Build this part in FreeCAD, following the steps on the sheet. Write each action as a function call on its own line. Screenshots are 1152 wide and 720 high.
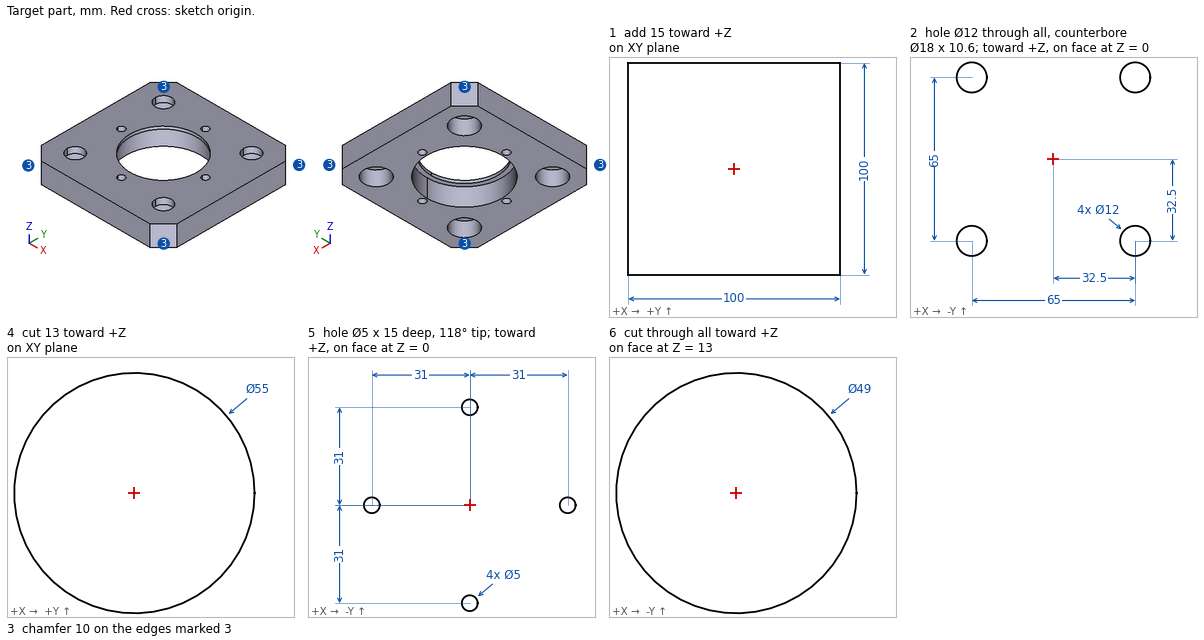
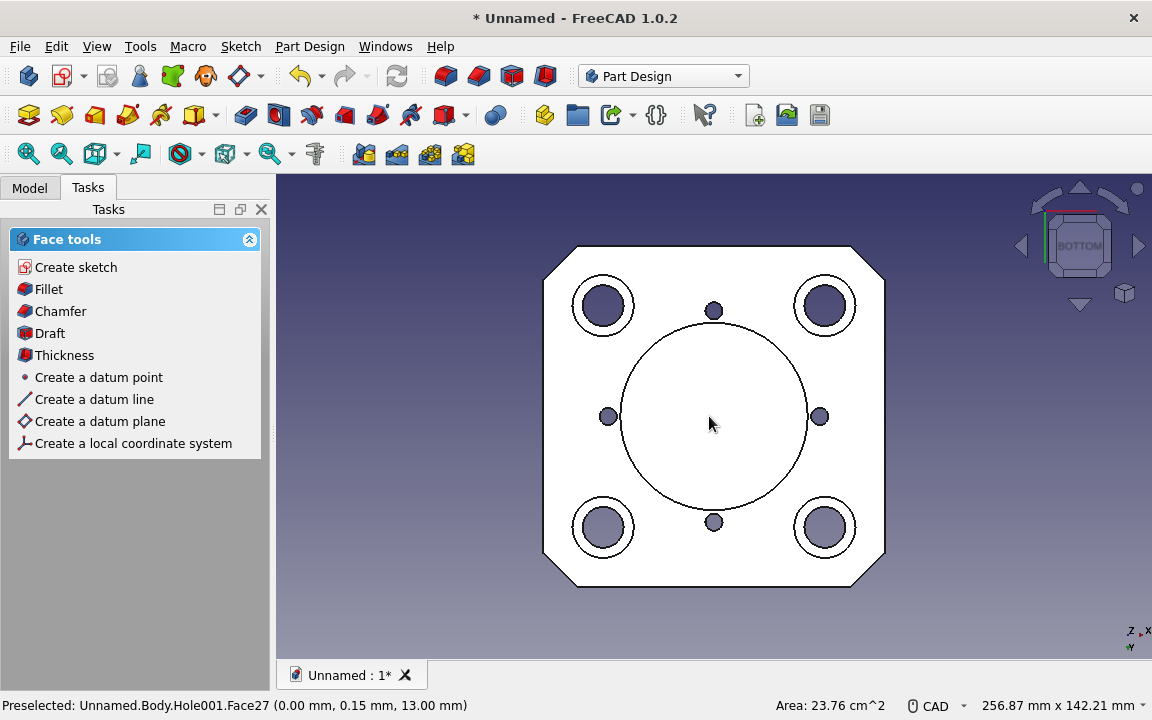
click(62, 76)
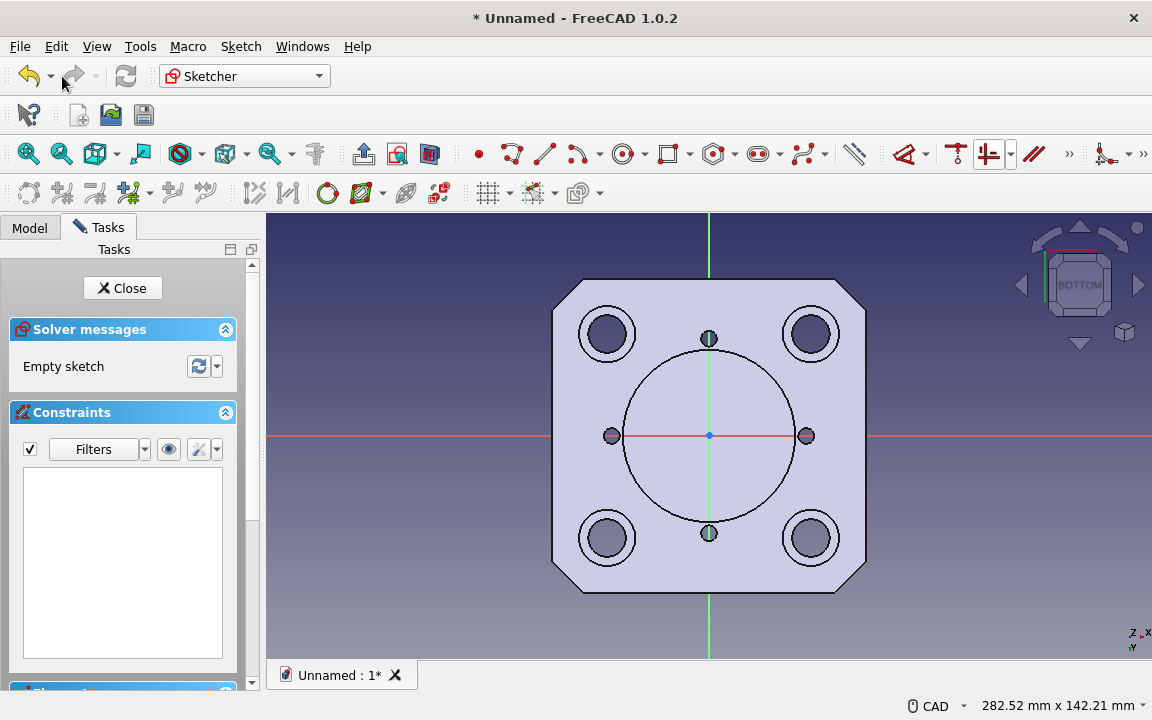
click(430, 154)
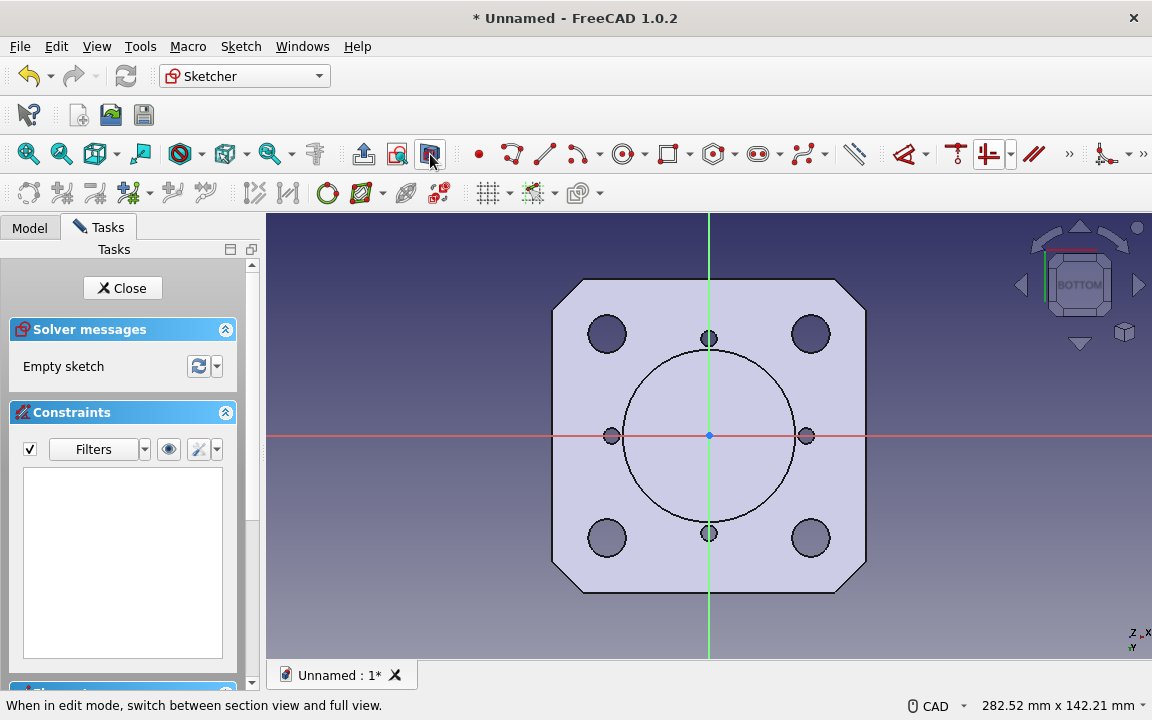
scroll(792, 436, up, 3)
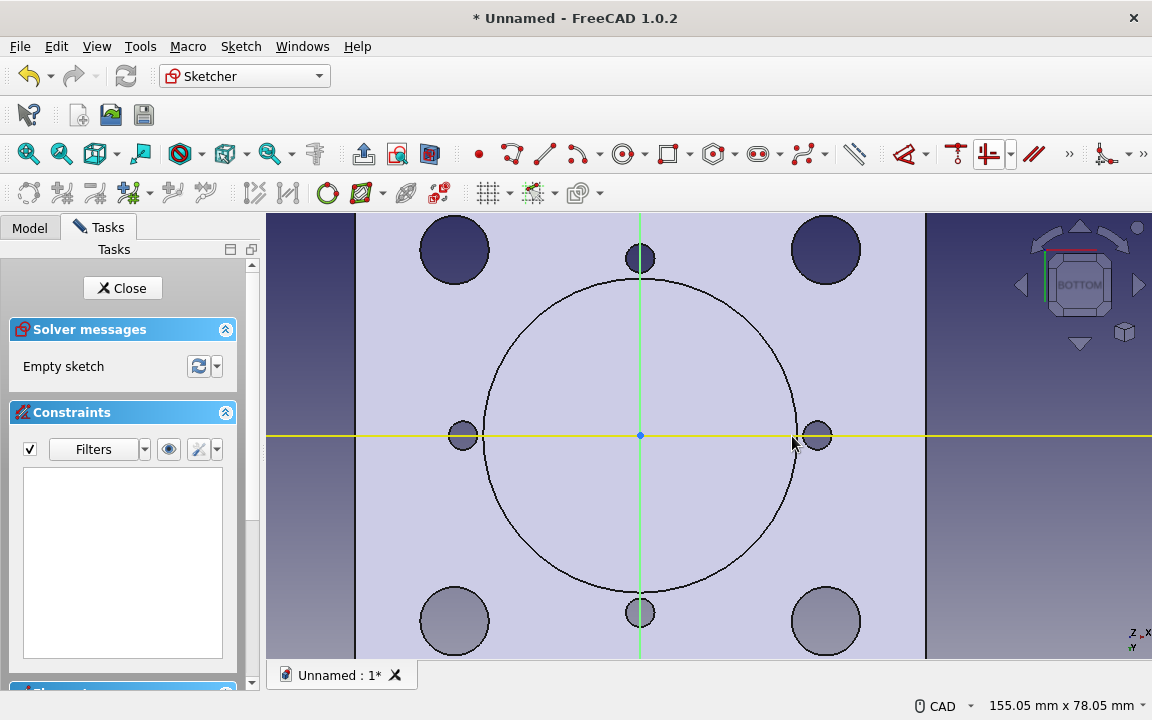
click(622, 154)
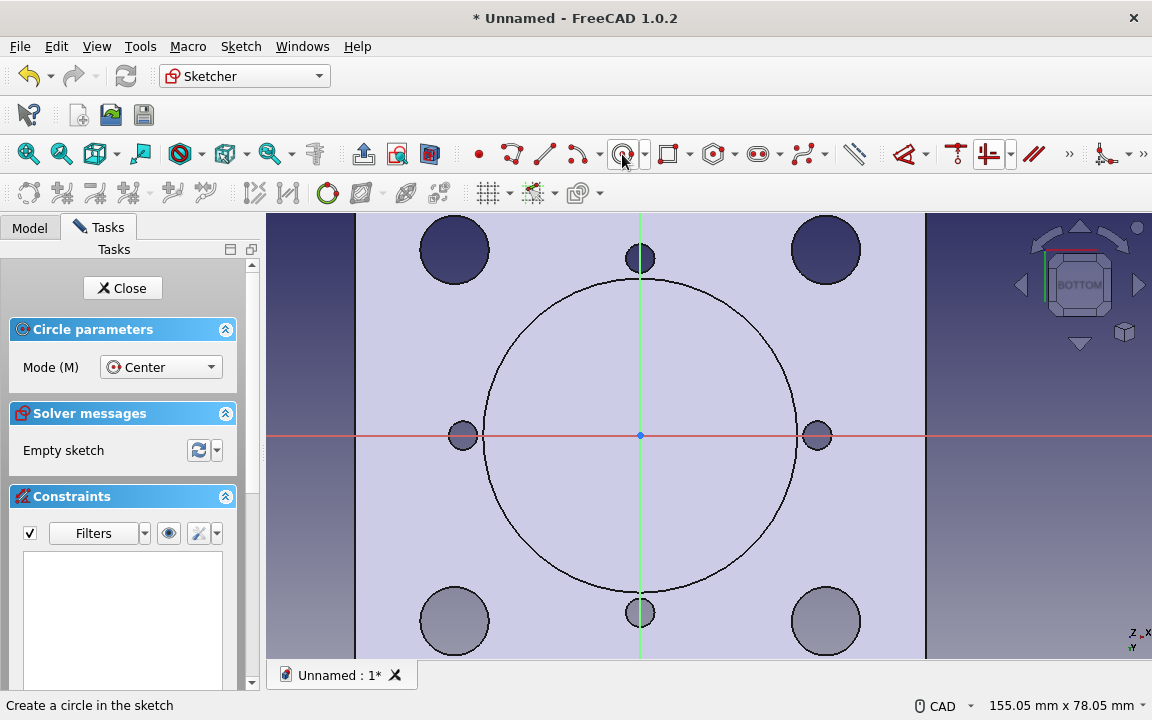
click(640, 436)
move(739, 337)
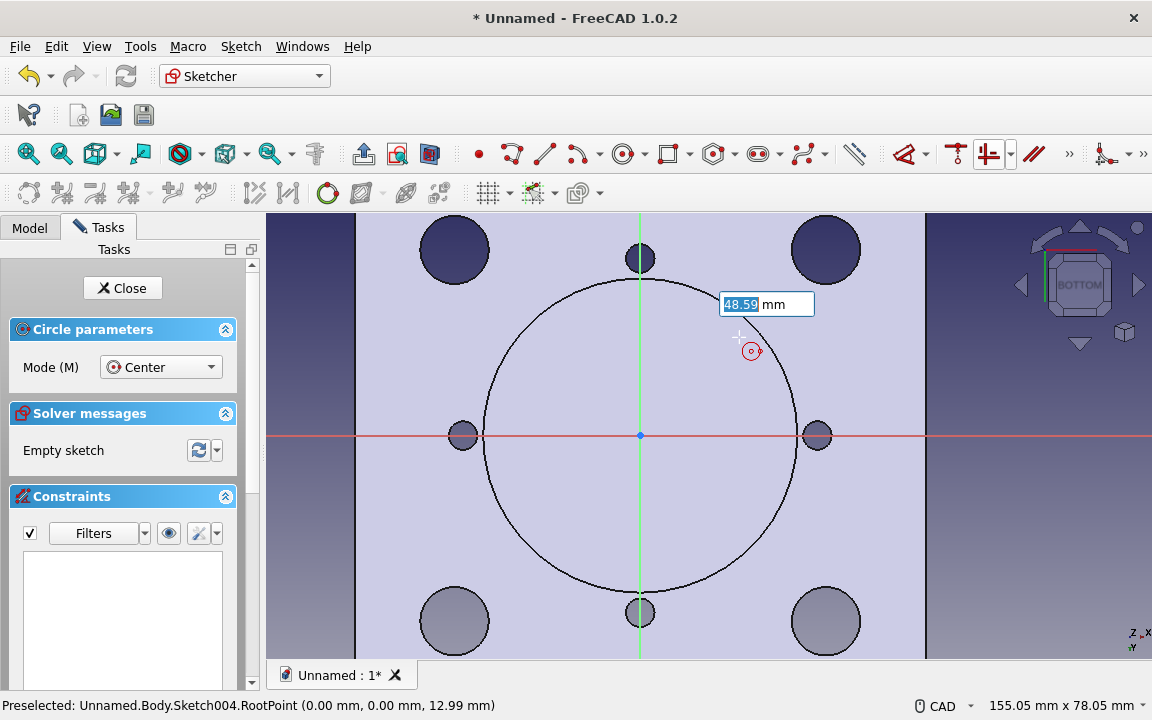
text(49)
key(Return)
key(Escape)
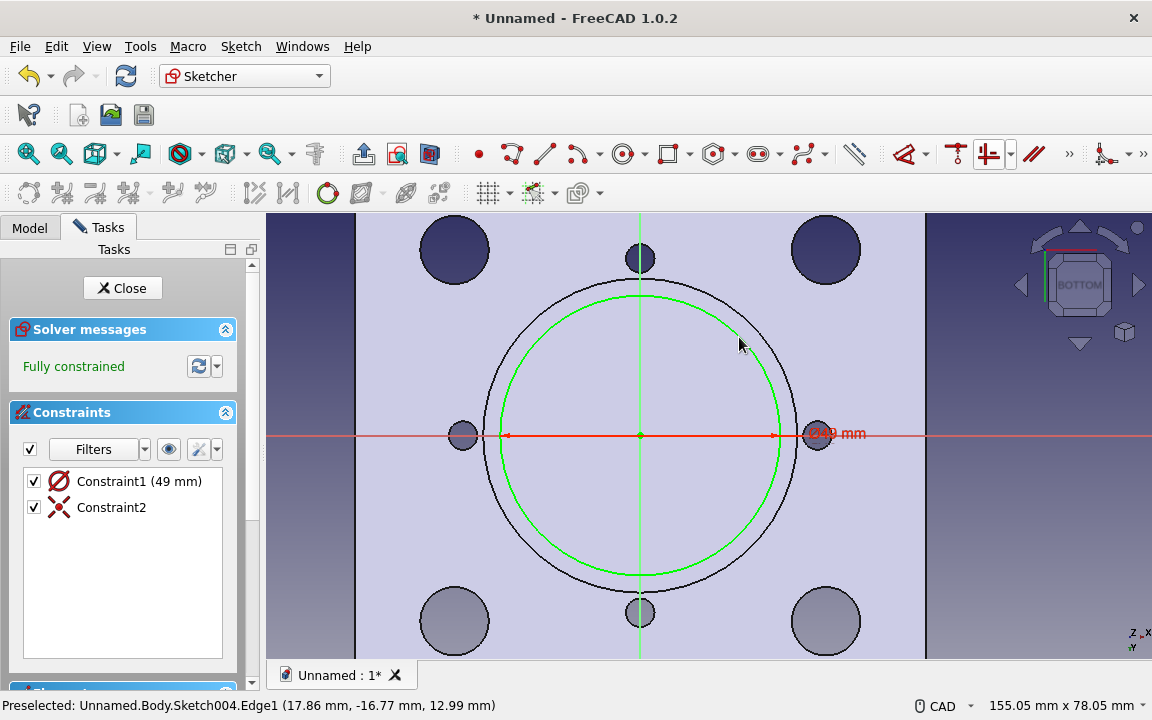
click(123, 288)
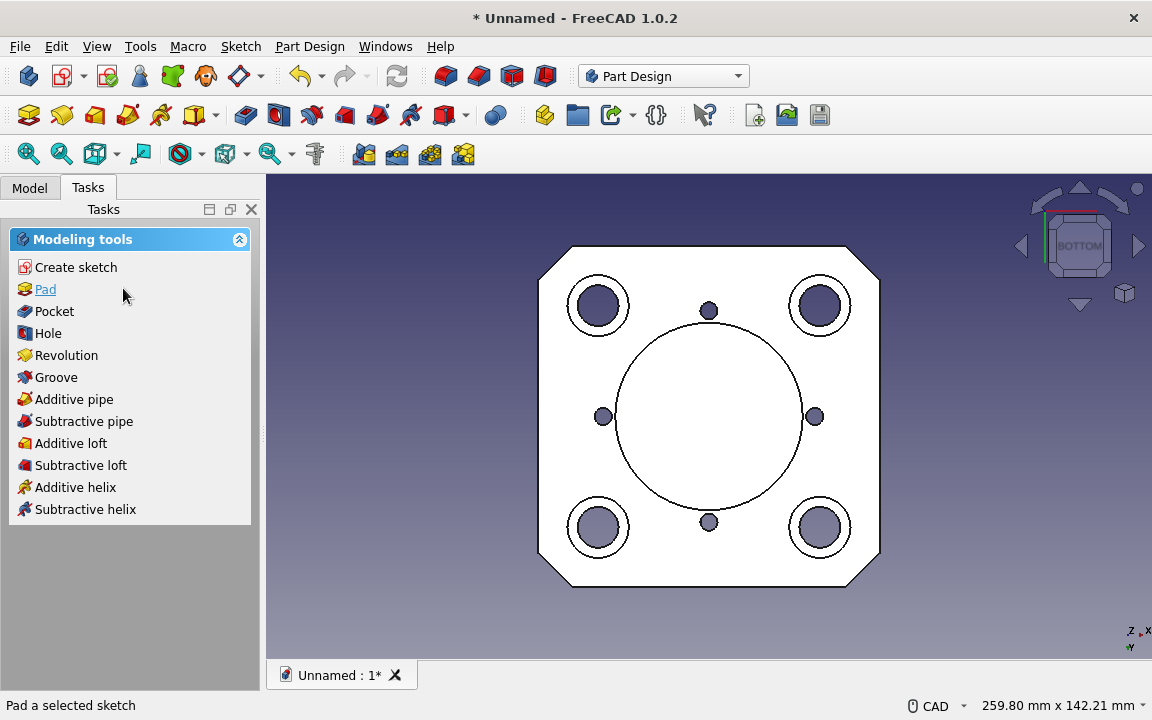
click(246, 116)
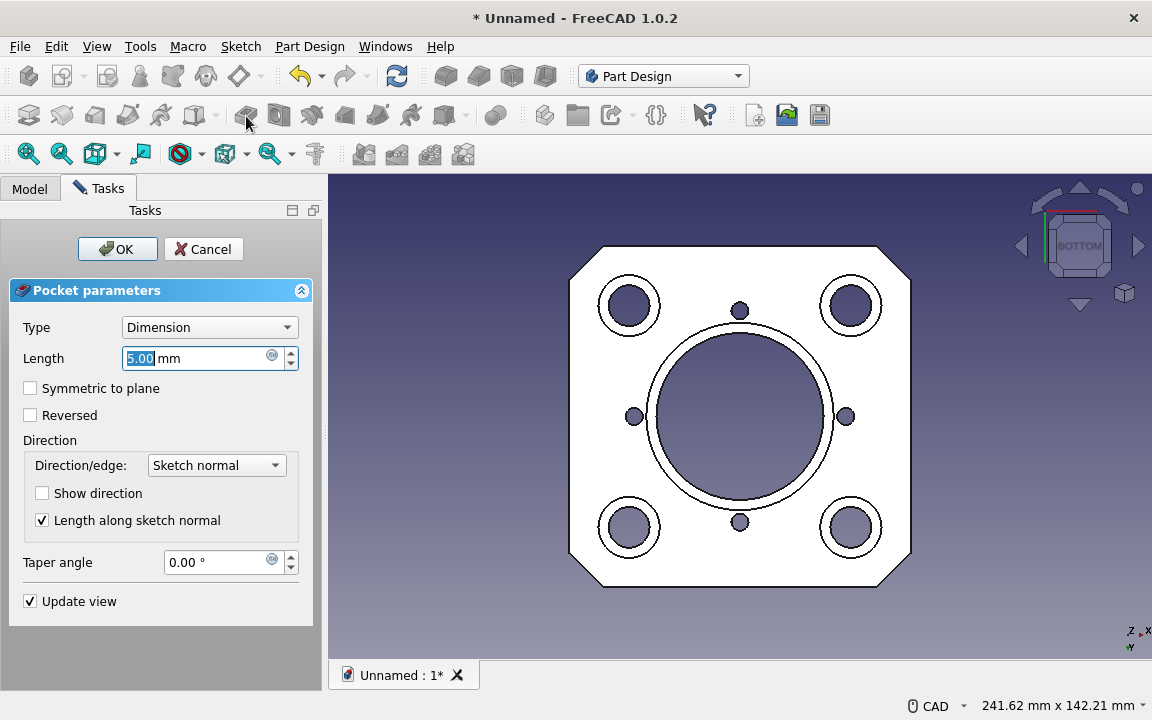
click(210, 328)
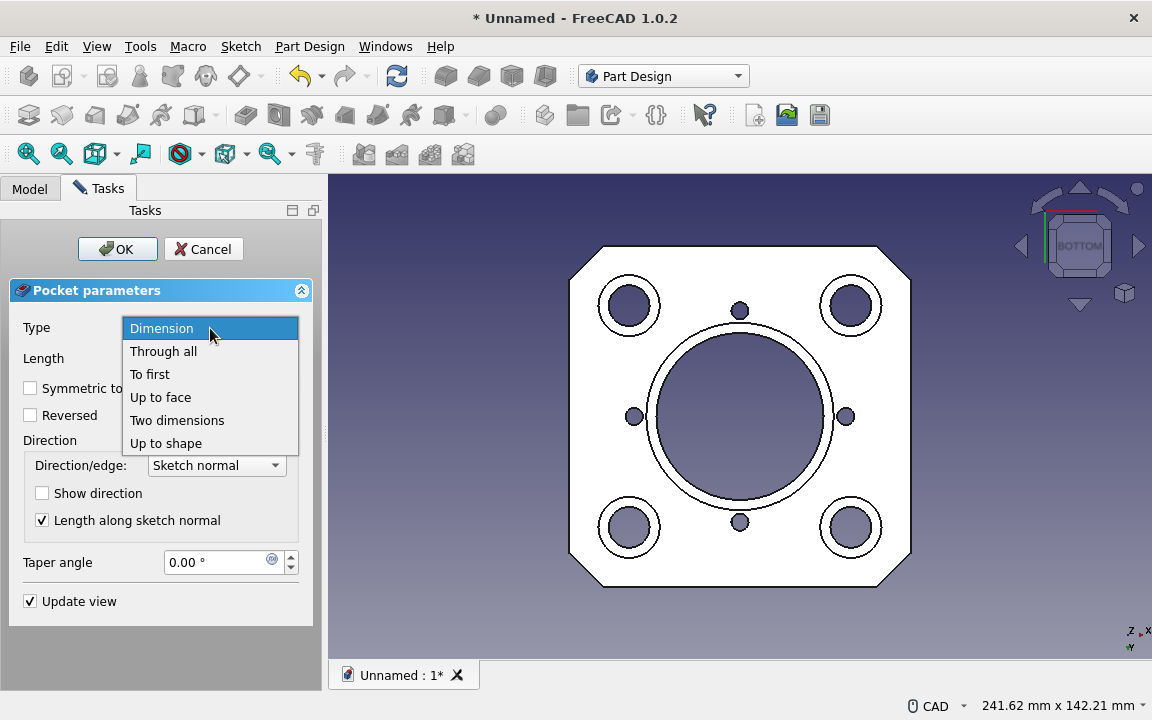
click(208, 352)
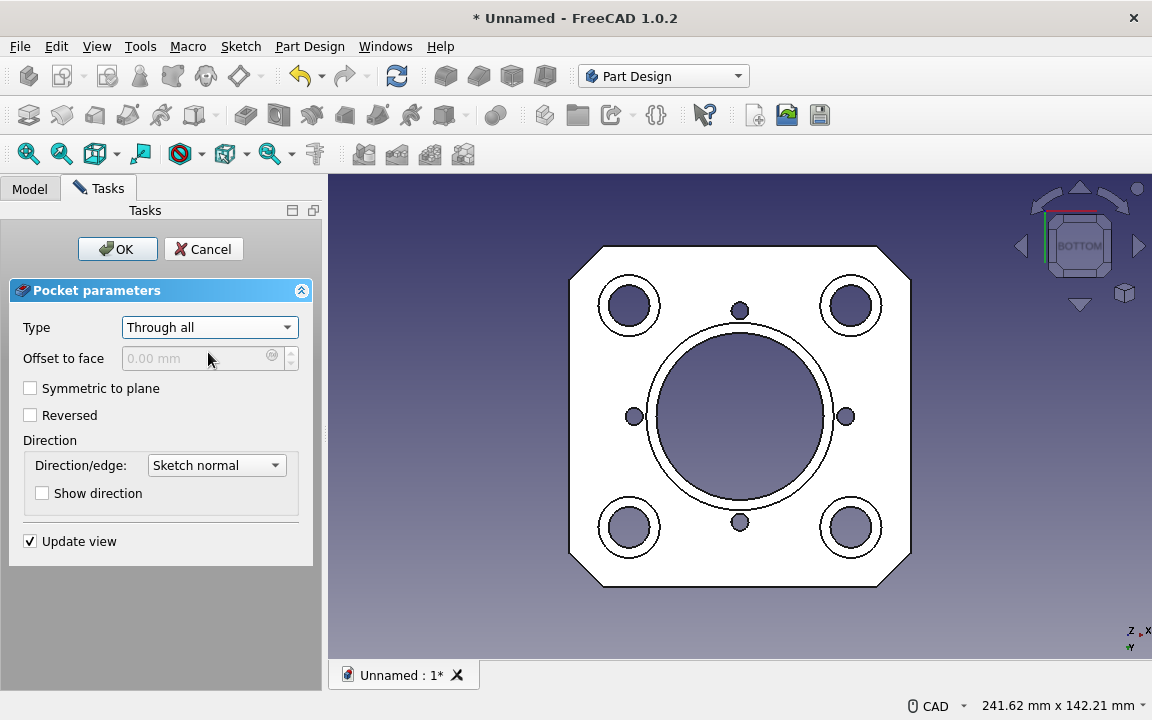
click(118, 249)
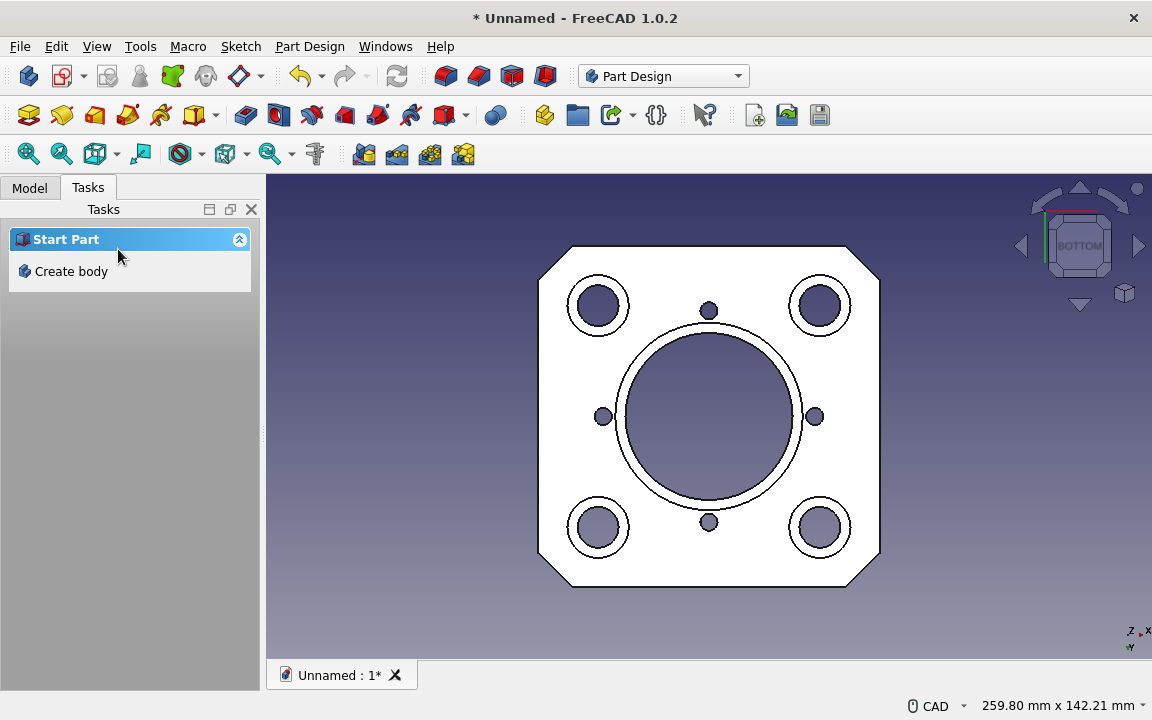
key(0)